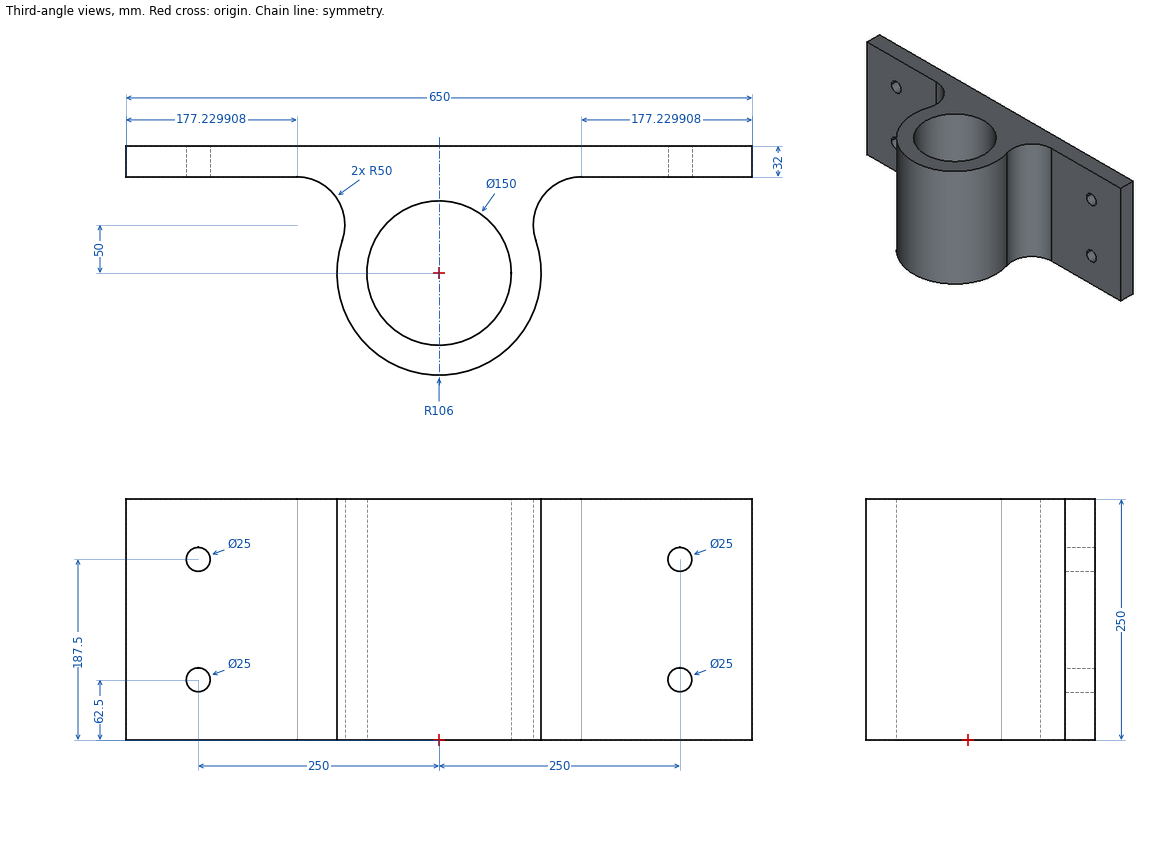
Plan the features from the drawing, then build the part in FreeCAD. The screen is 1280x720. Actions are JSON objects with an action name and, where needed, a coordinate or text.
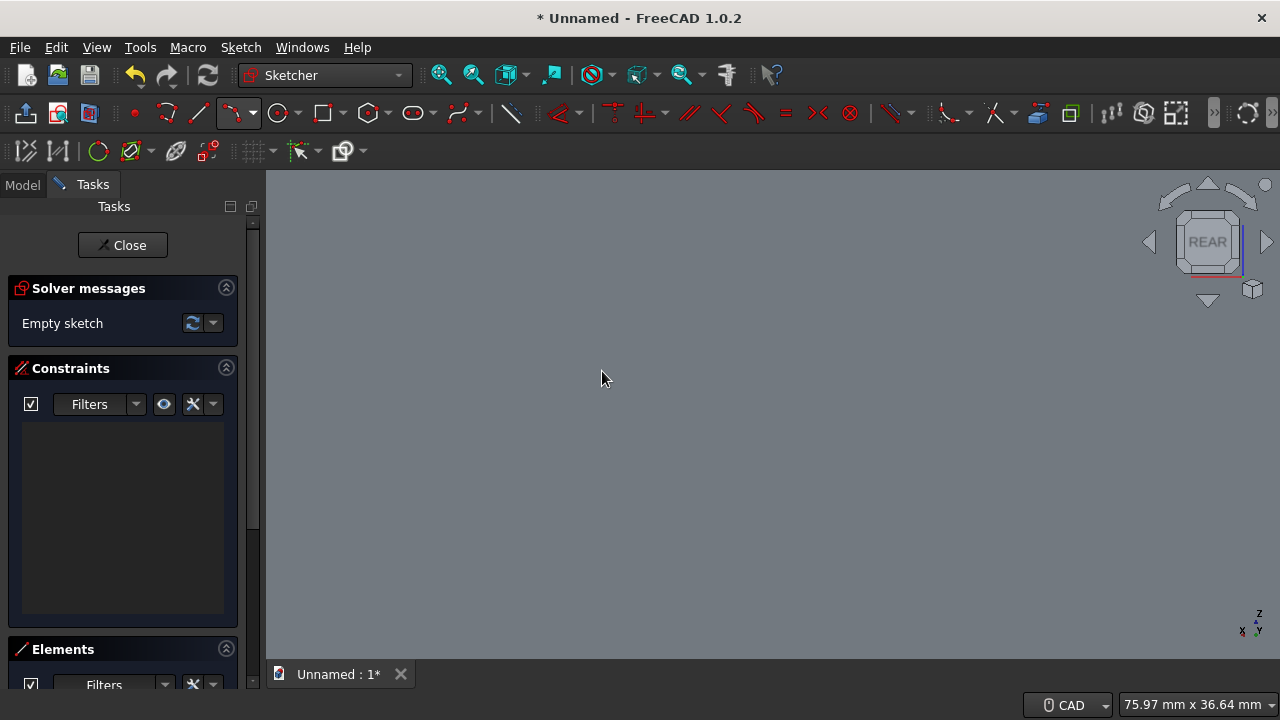
{"action": "left_click", "coordinate": [278, 114]}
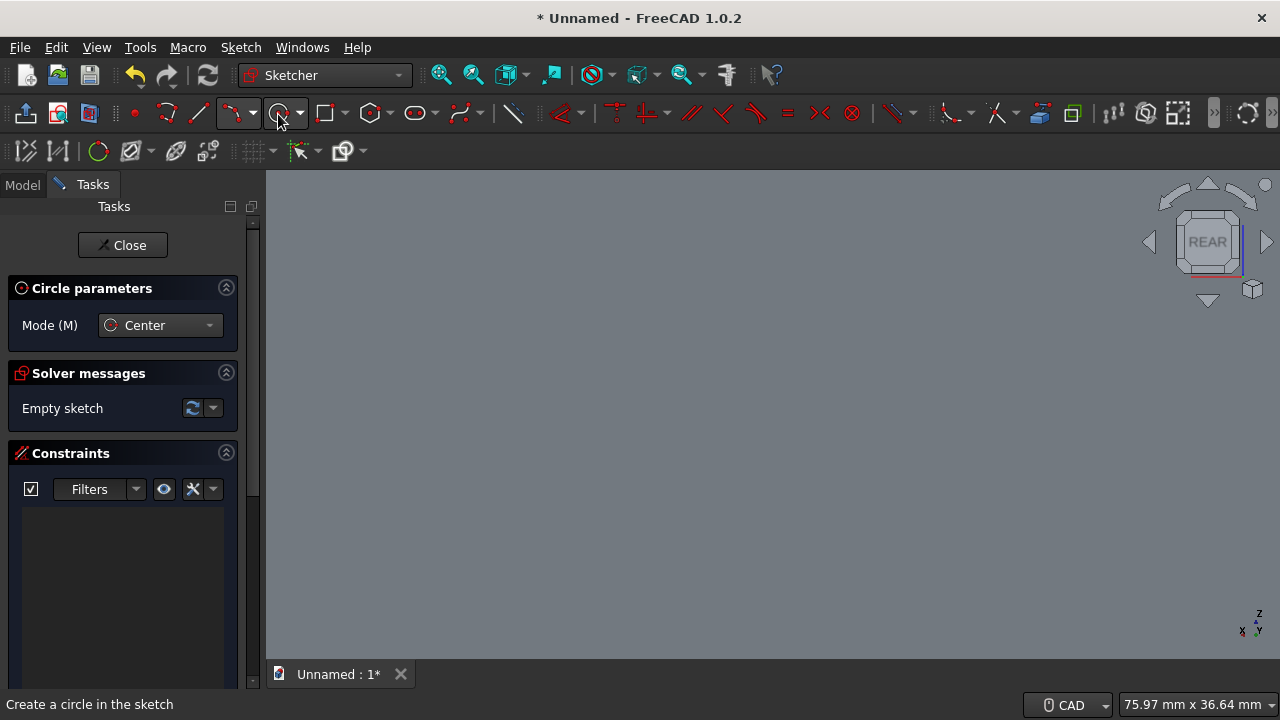
{"action": "left_click", "coordinate": [693, 403]}
{"action": "mouse_move", "coordinate": [811, 285]}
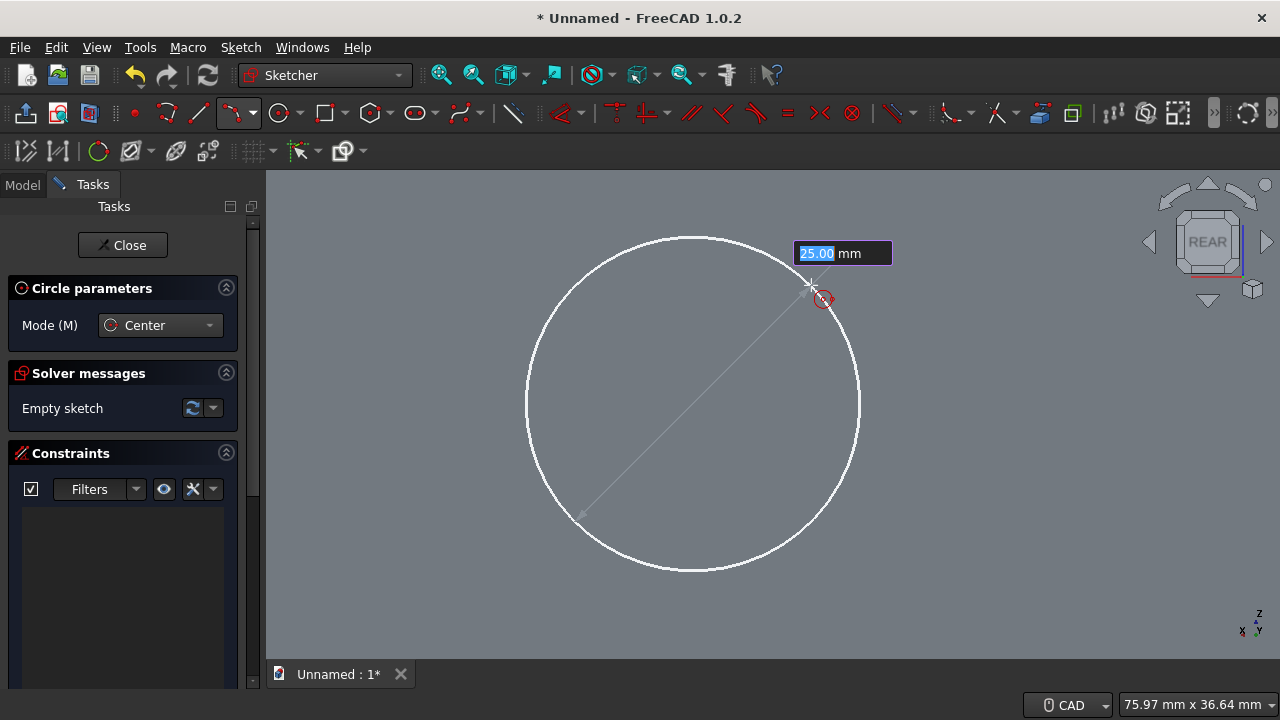
{"action": "type", "text": "25"}
{"action": "key", "text": "Return"}
{"action": "key", "text": "Escape"}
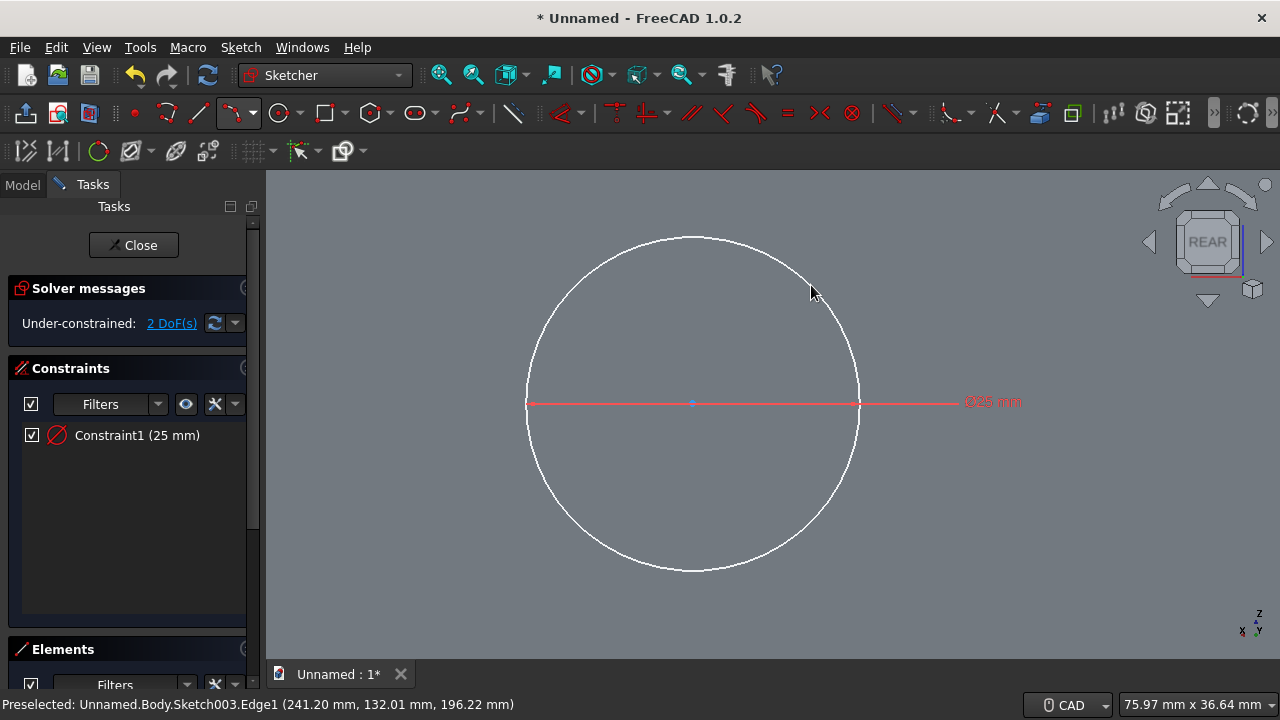
{"action": "left_click", "coordinate": [560, 114]}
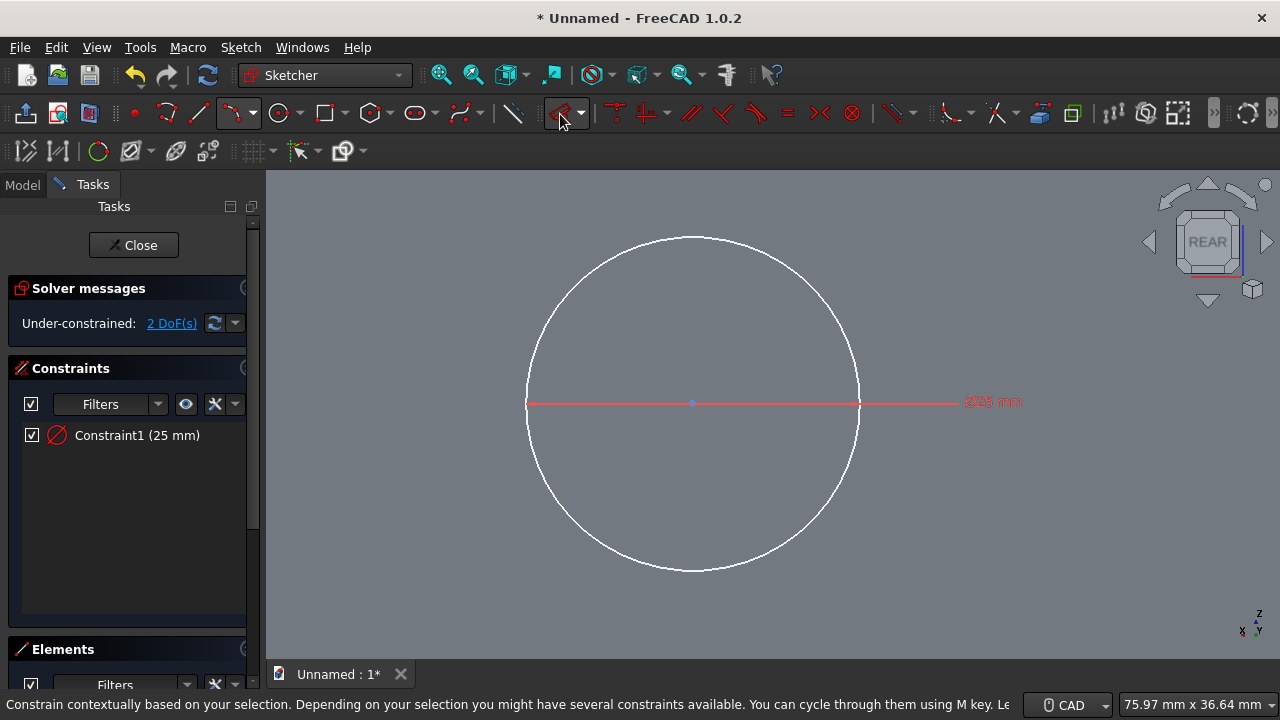
{"action": "left_click", "coordinate": [693, 404]}
{"action": "left_click", "coordinate": [904, 370]}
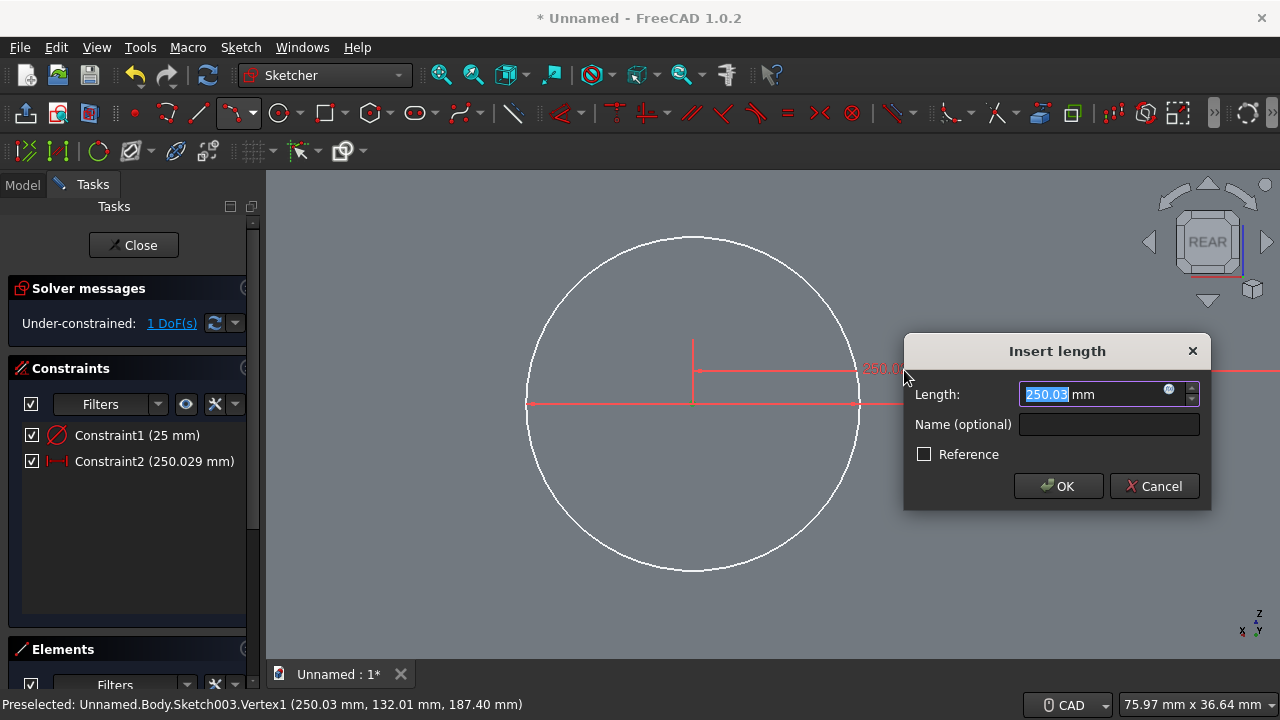
{"action": "type", "text": "250"}
{"action": "key", "text": "Return"}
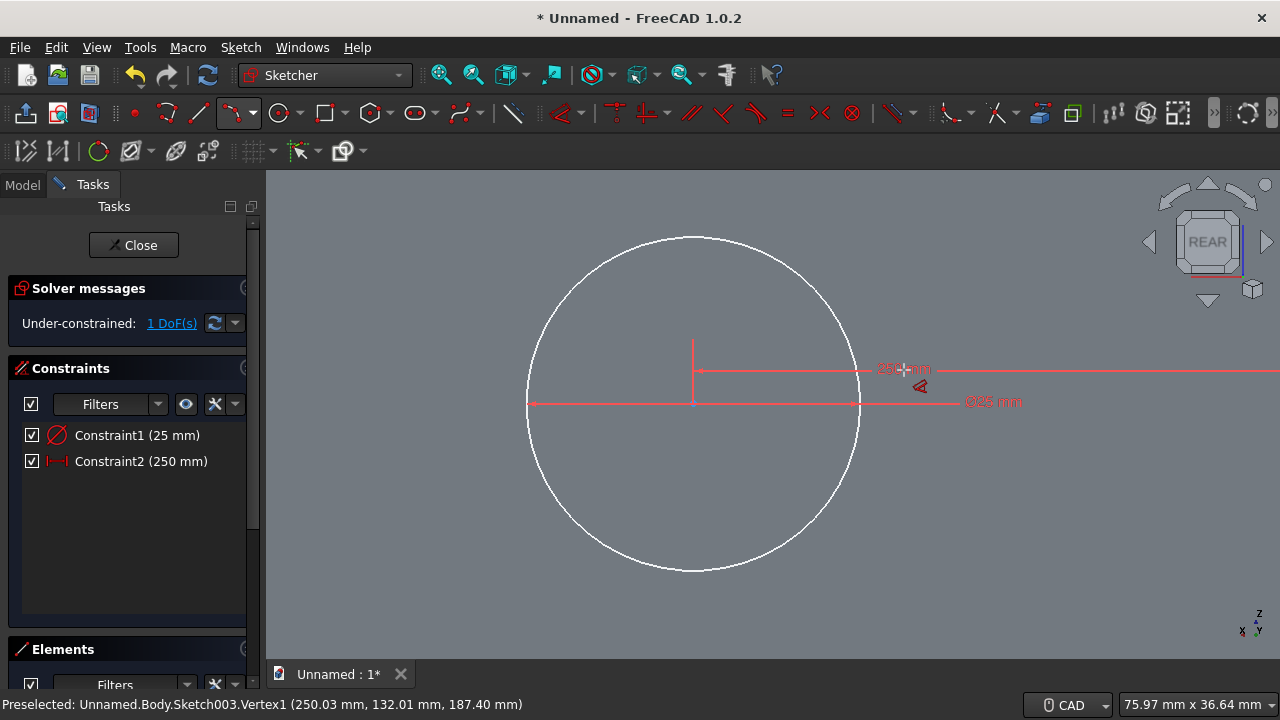
{"action": "left_click", "coordinate": [693, 404]}
{"action": "left_click", "coordinate": [659, 518]}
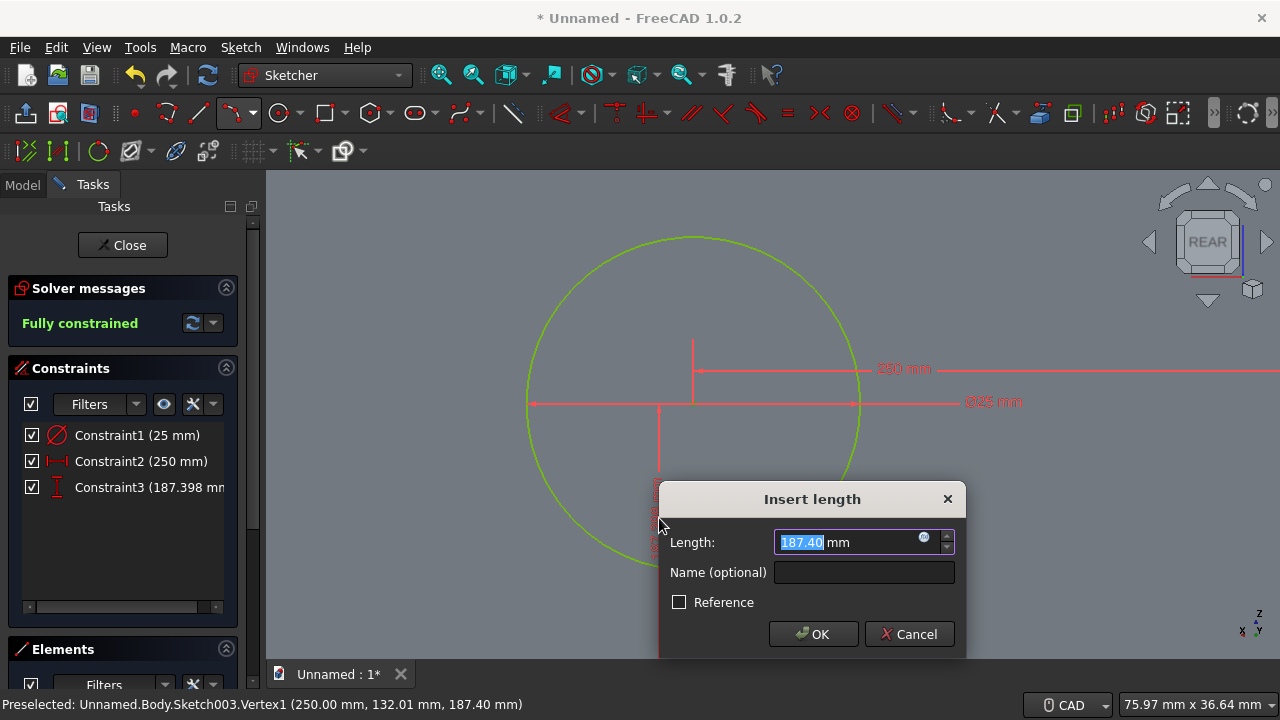
{"action": "type", "text": "187.5"}
{"action": "key", "text": "Return"}
{"action": "key", "text": "Escape"}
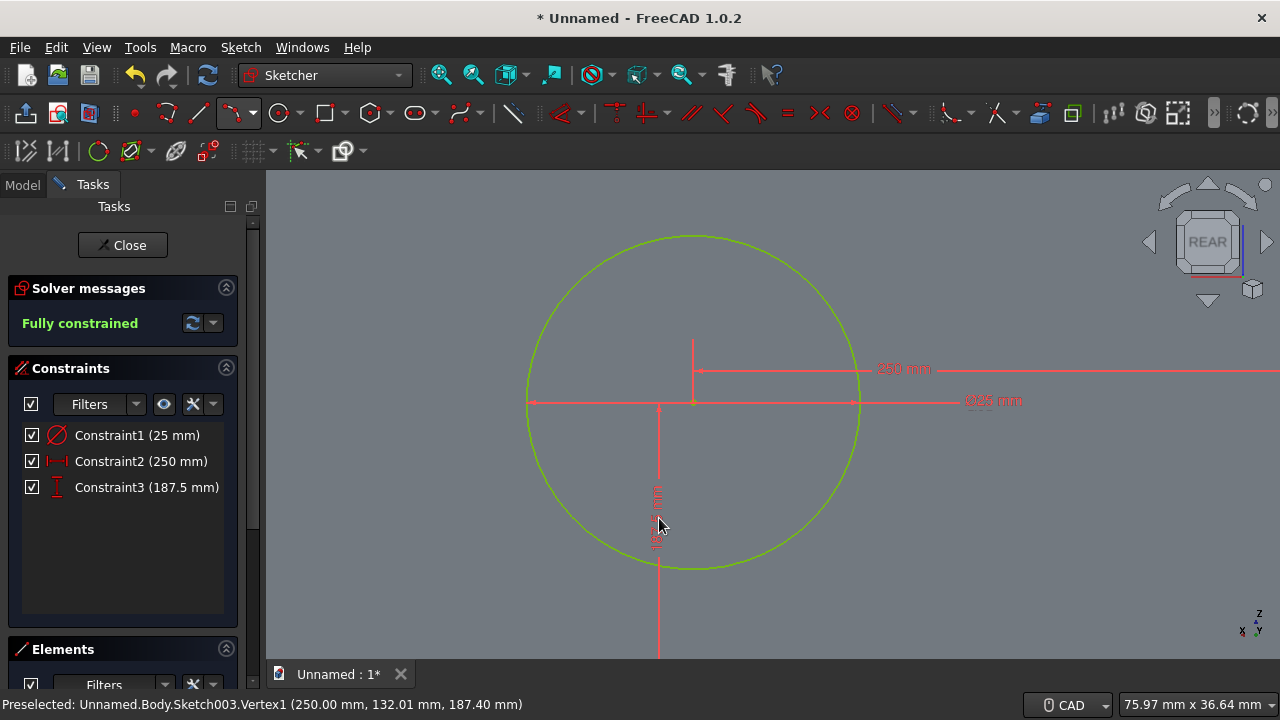
{"action": "left_click", "coordinate": [123, 245]}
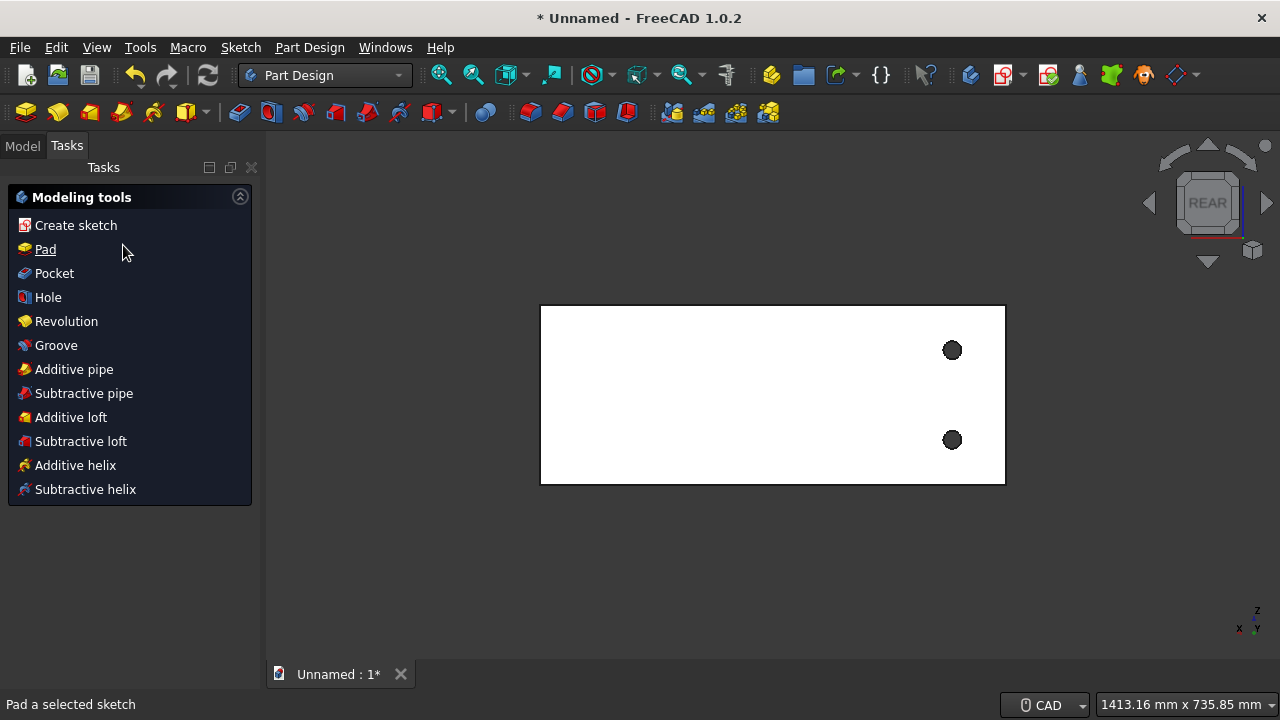
{"action": "left_click", "coordinate": [240, 112]}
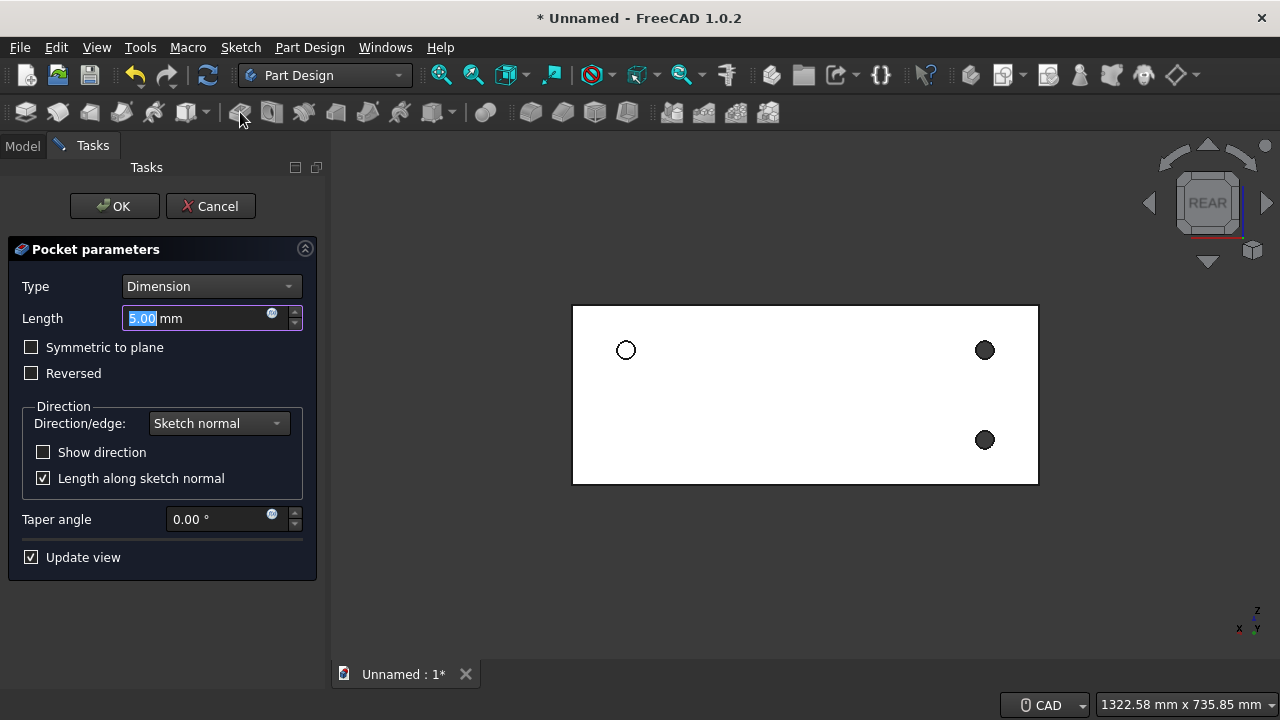
{"action": "left_click", "coordinate": [212, 286]}